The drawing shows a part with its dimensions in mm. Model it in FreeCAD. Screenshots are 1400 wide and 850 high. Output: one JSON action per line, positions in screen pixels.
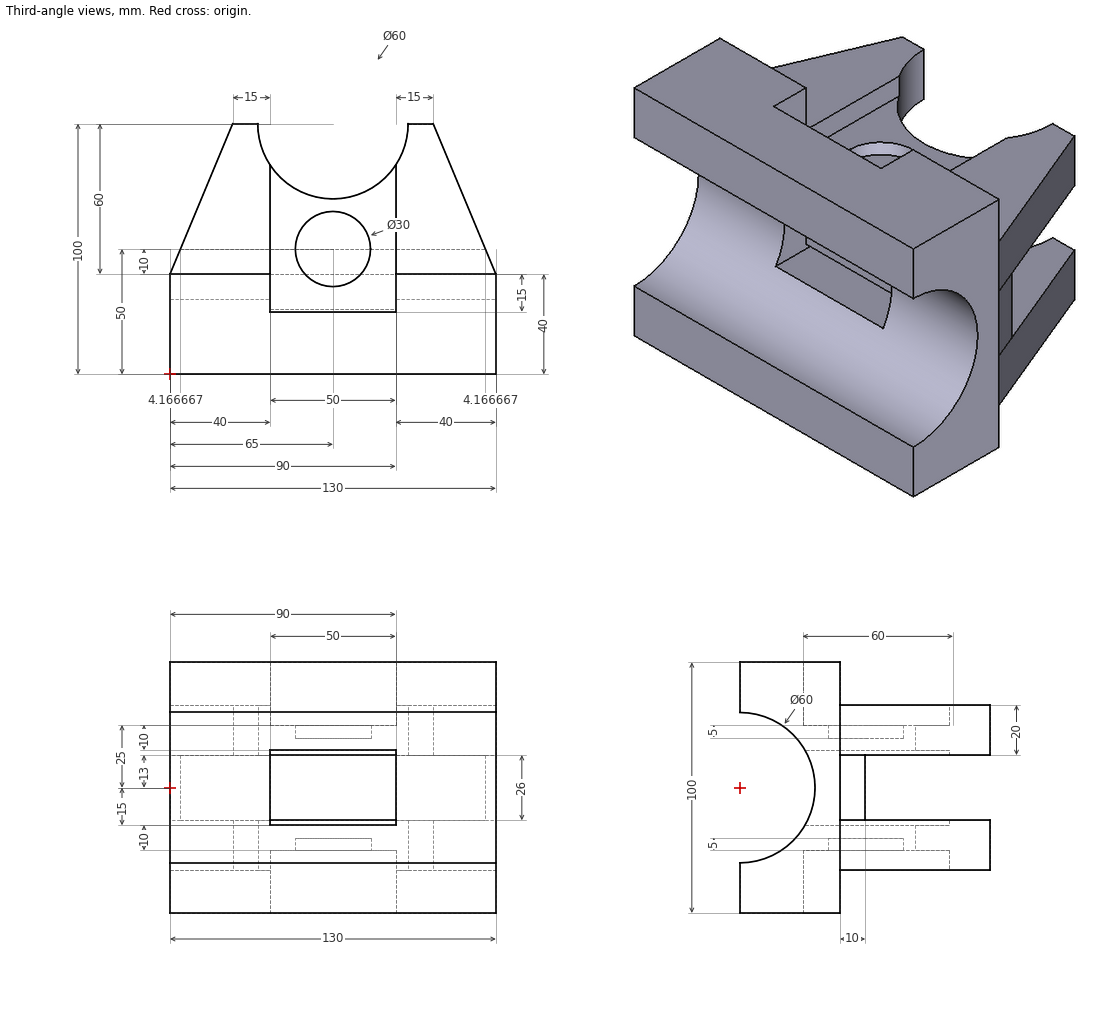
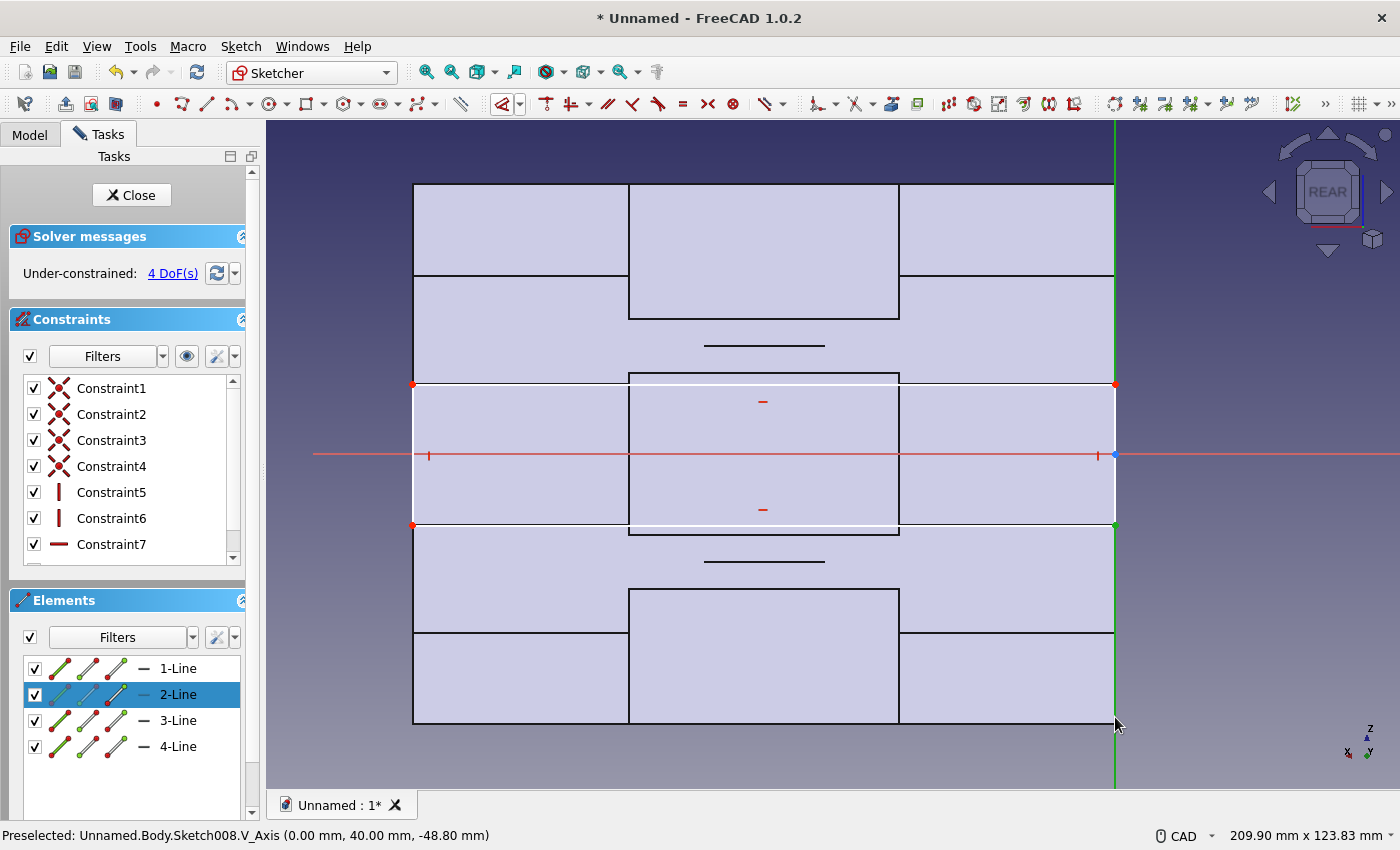
{"action": "left_click", "coordinate": [546, 104]}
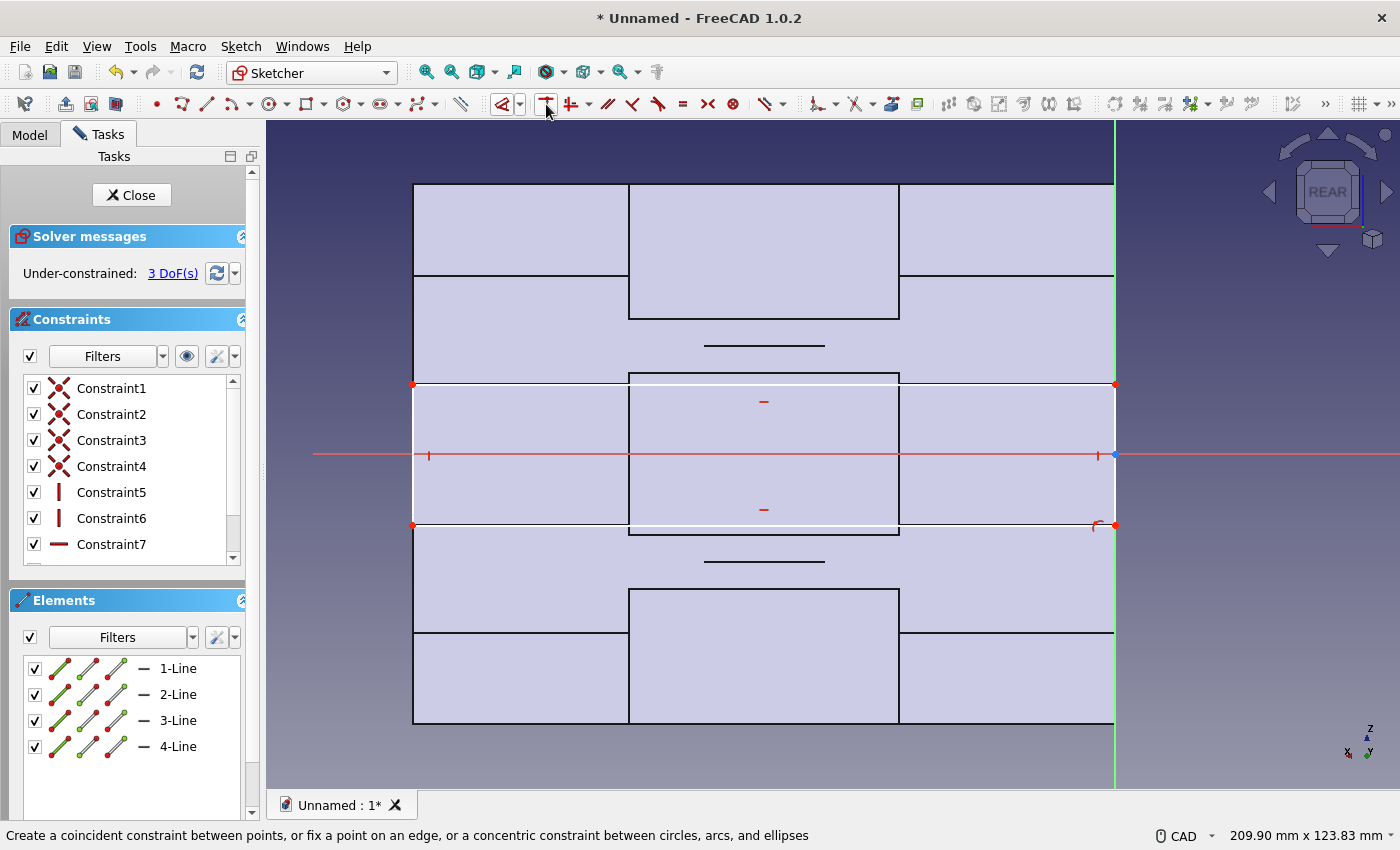
{"action": "left_click", "coordinate": [413, 427]}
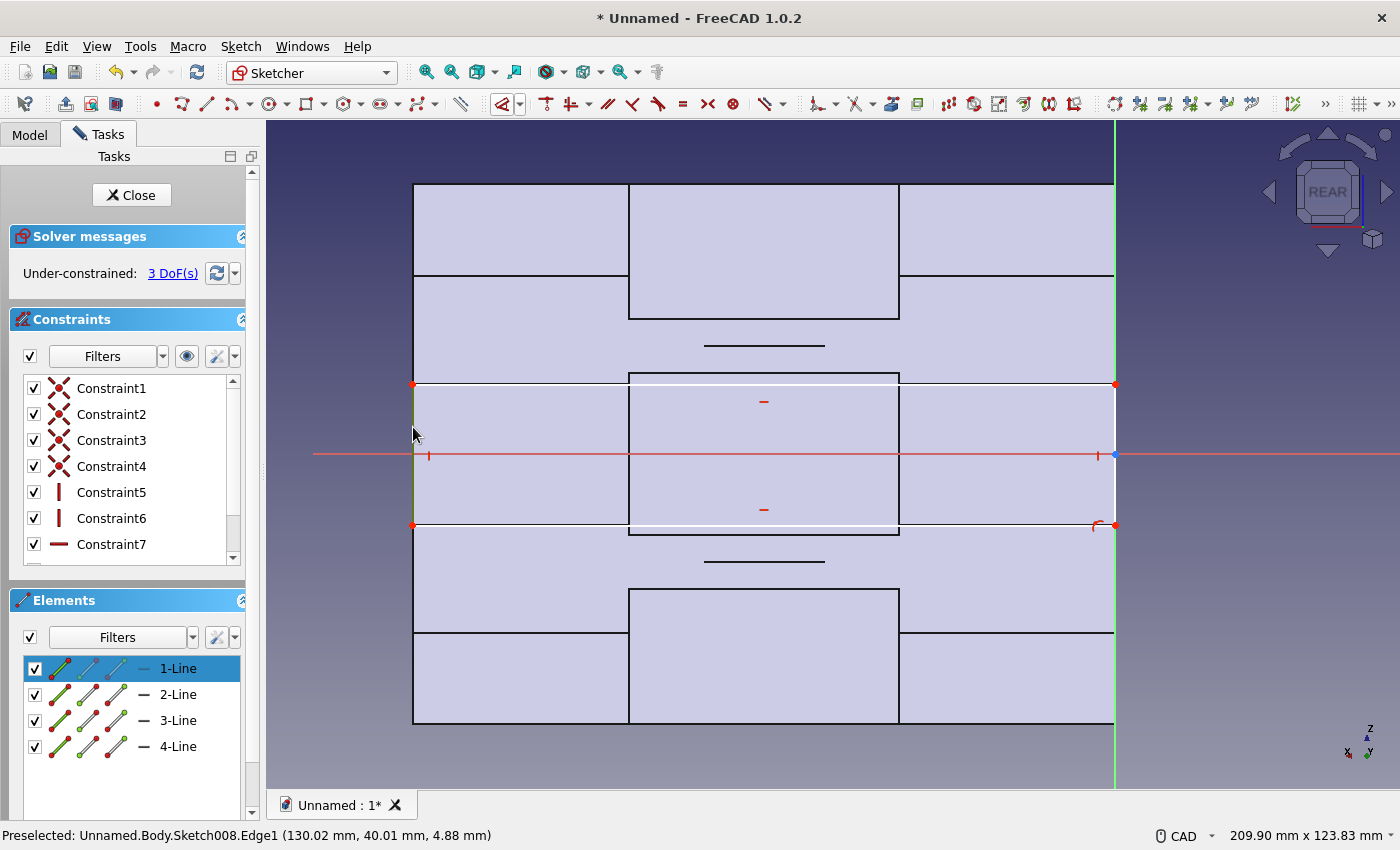
{"action": "key", "text": "i"}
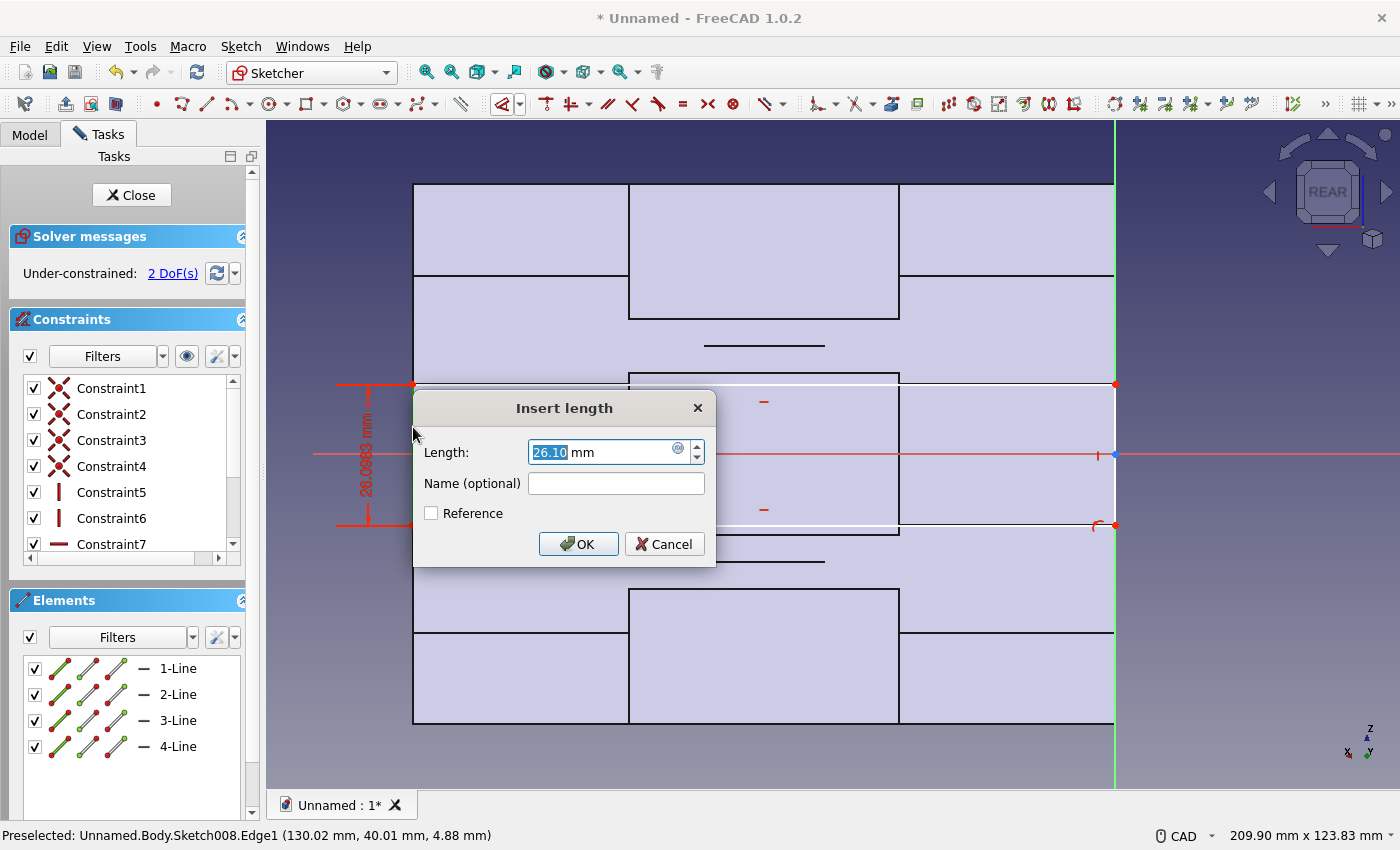
{"action": "type", "text": "26"}
{"action": "key", "text": "Return"}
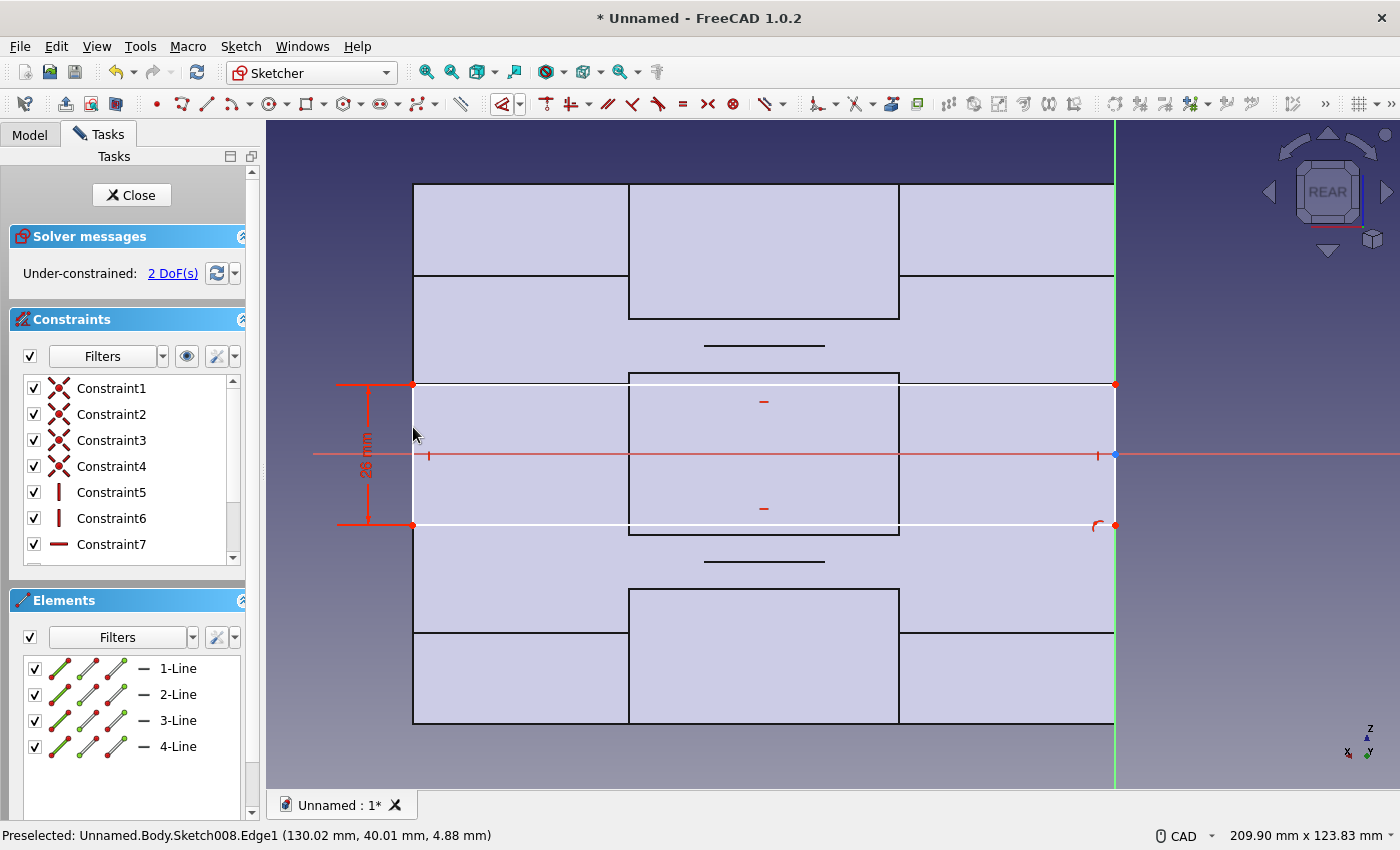
{"action": "left_click", "coordinate": [624, 525]}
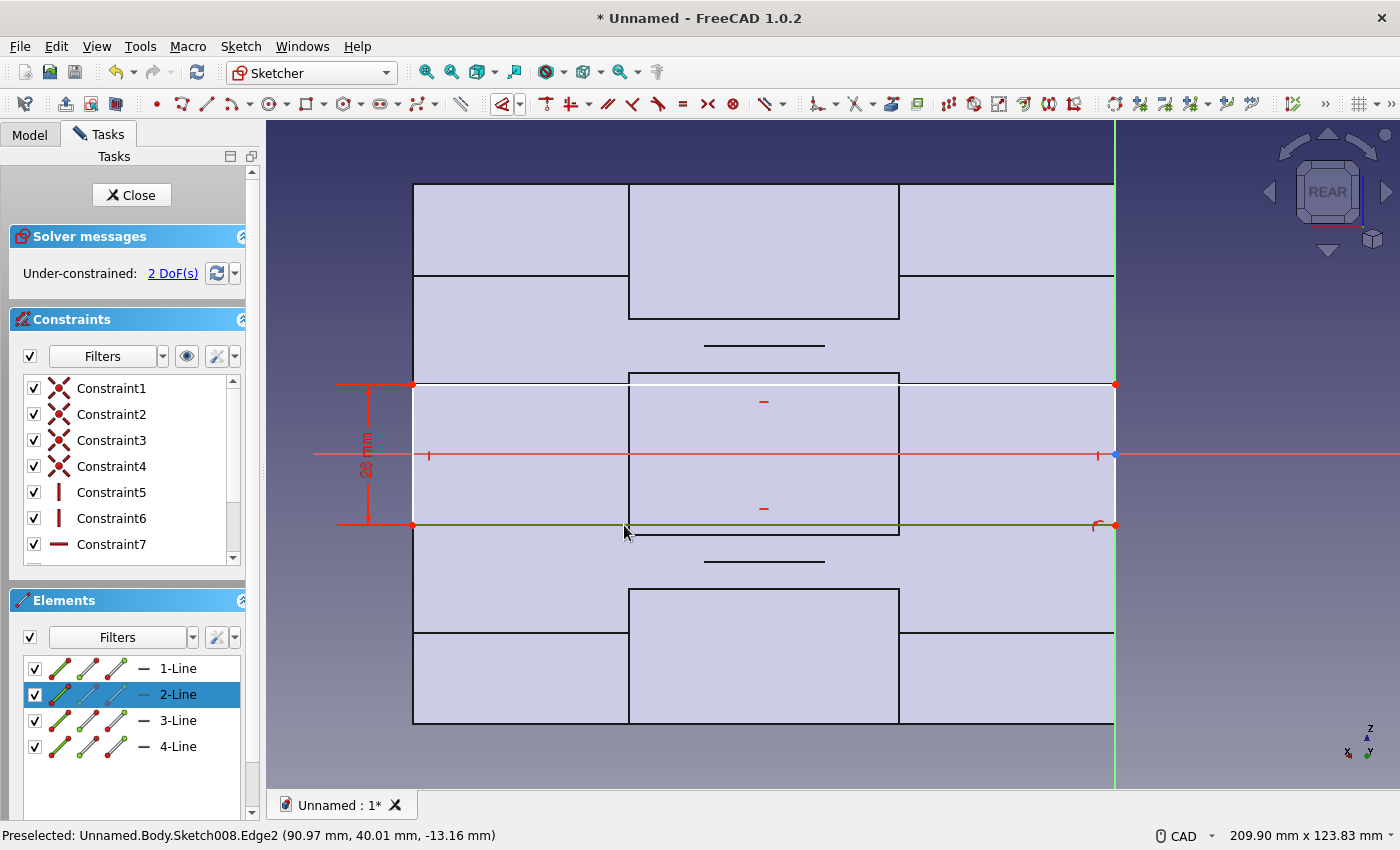
{"action": "key", "text": "l"}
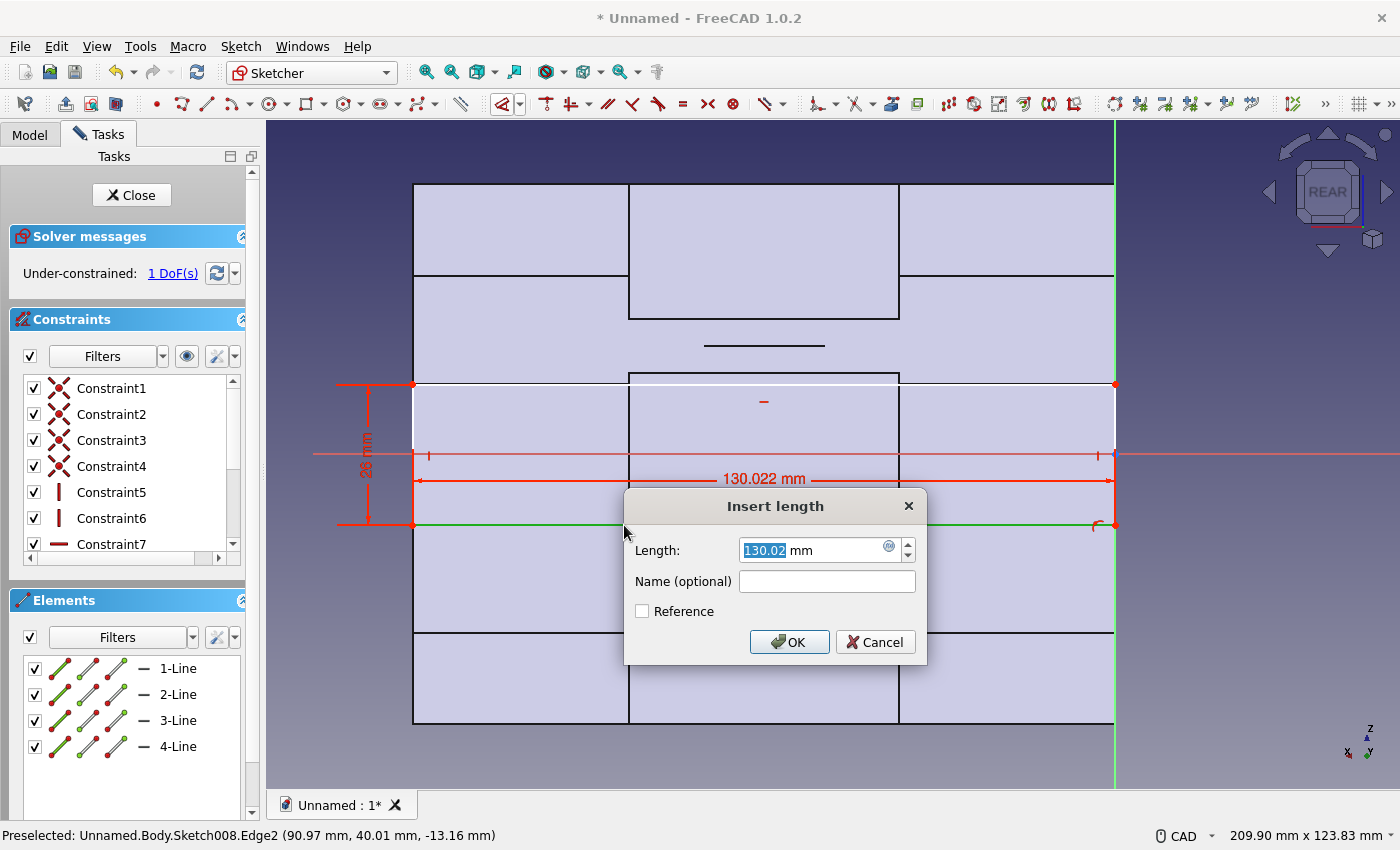
{"action": "type", "text": "130"}
{"action": "key", "text": "Return"}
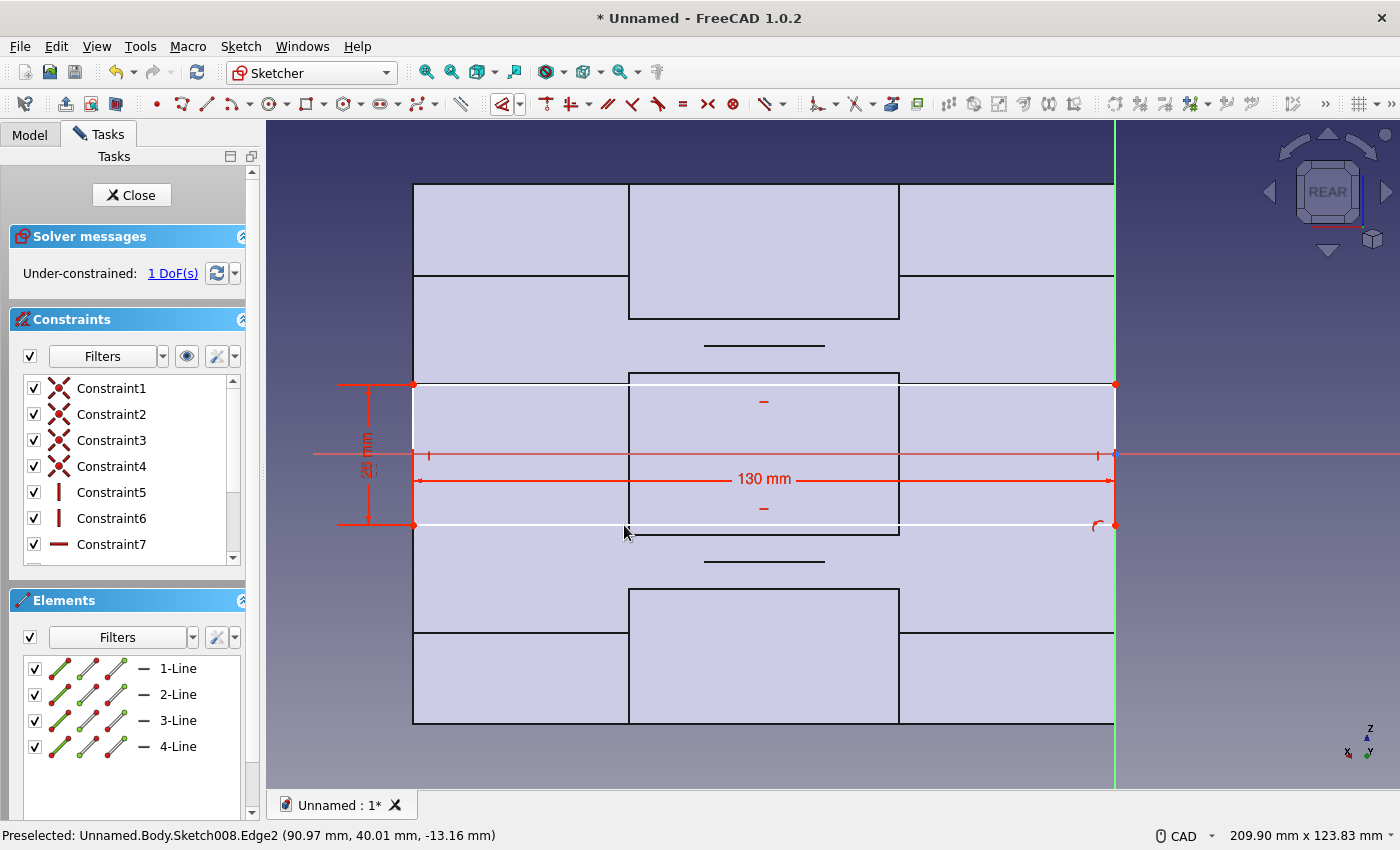
{"action": "left_click", "coordinate": [413, 385]}